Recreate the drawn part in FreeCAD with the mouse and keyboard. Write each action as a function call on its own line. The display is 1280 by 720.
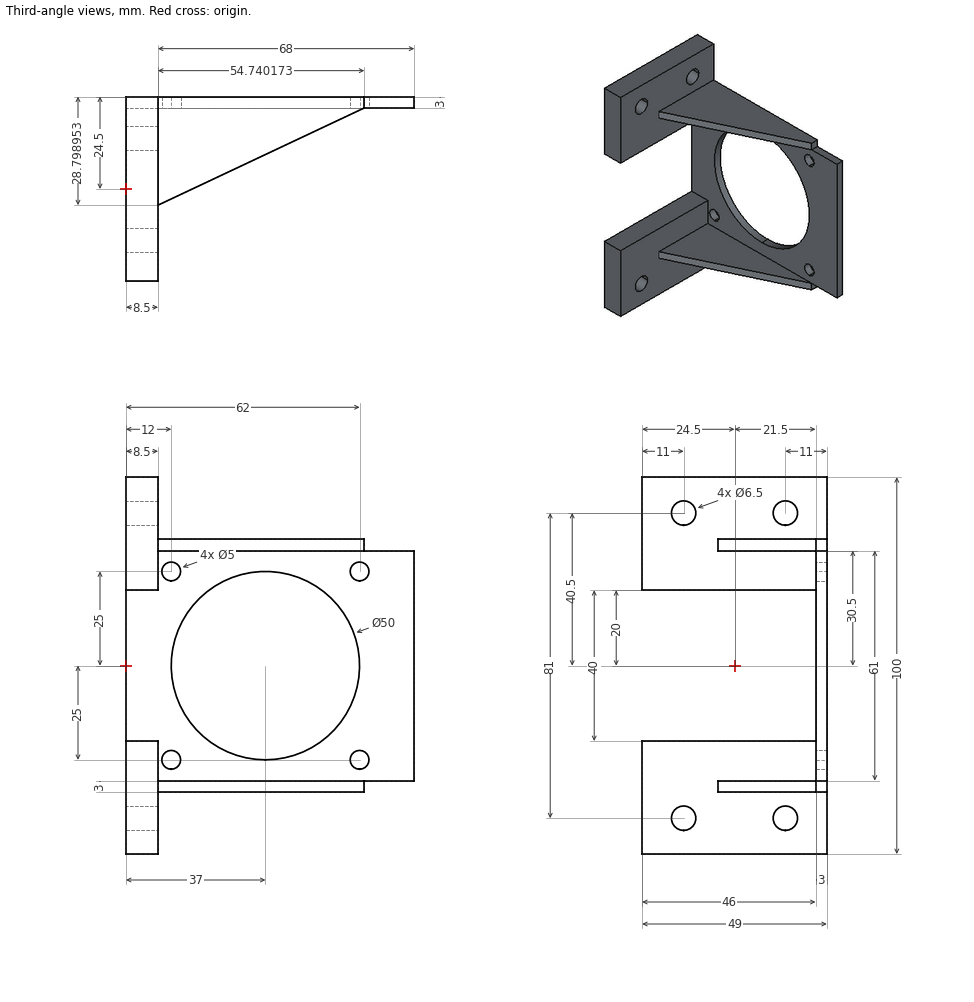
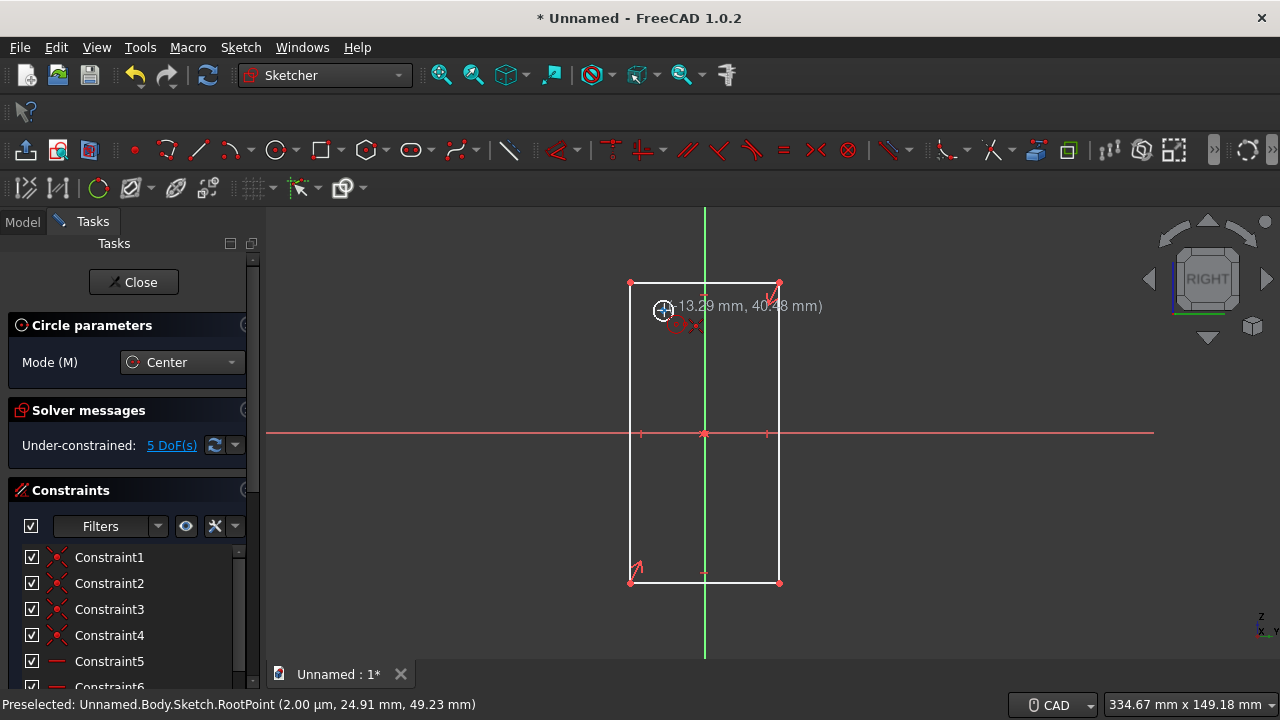
scroll(664, 556, up, 5)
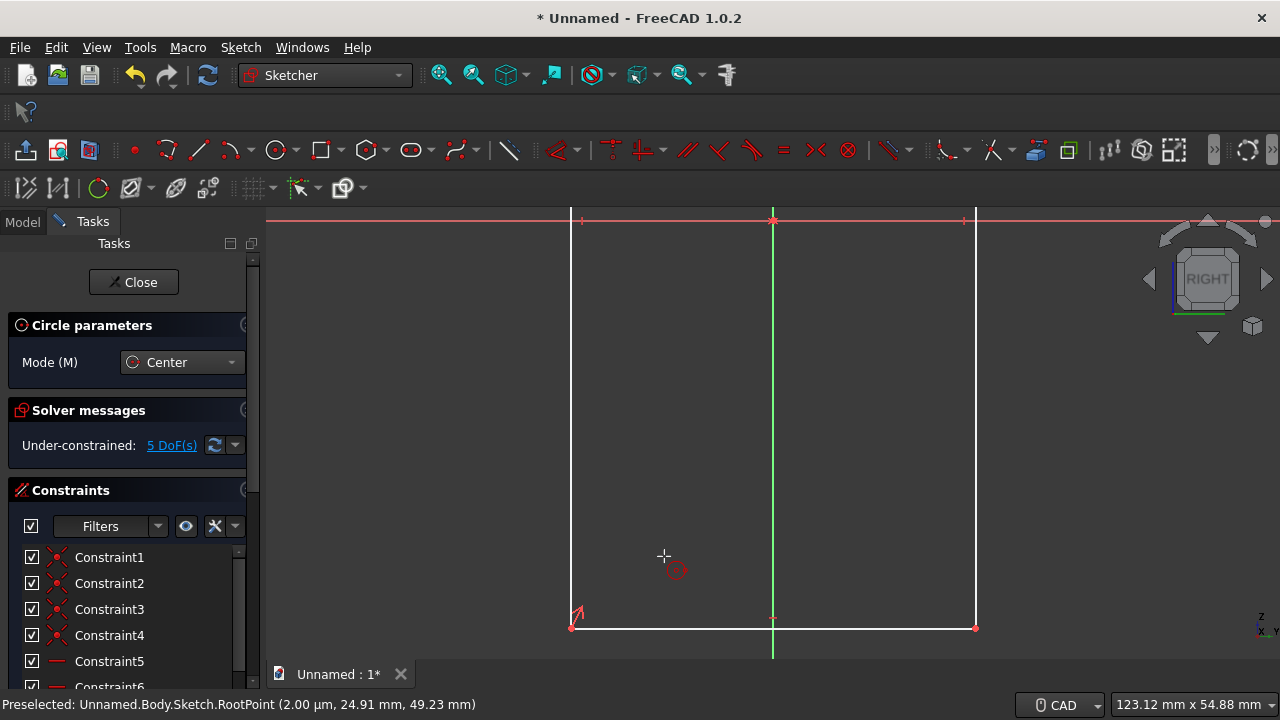
click(662, 554)
click(681, 535)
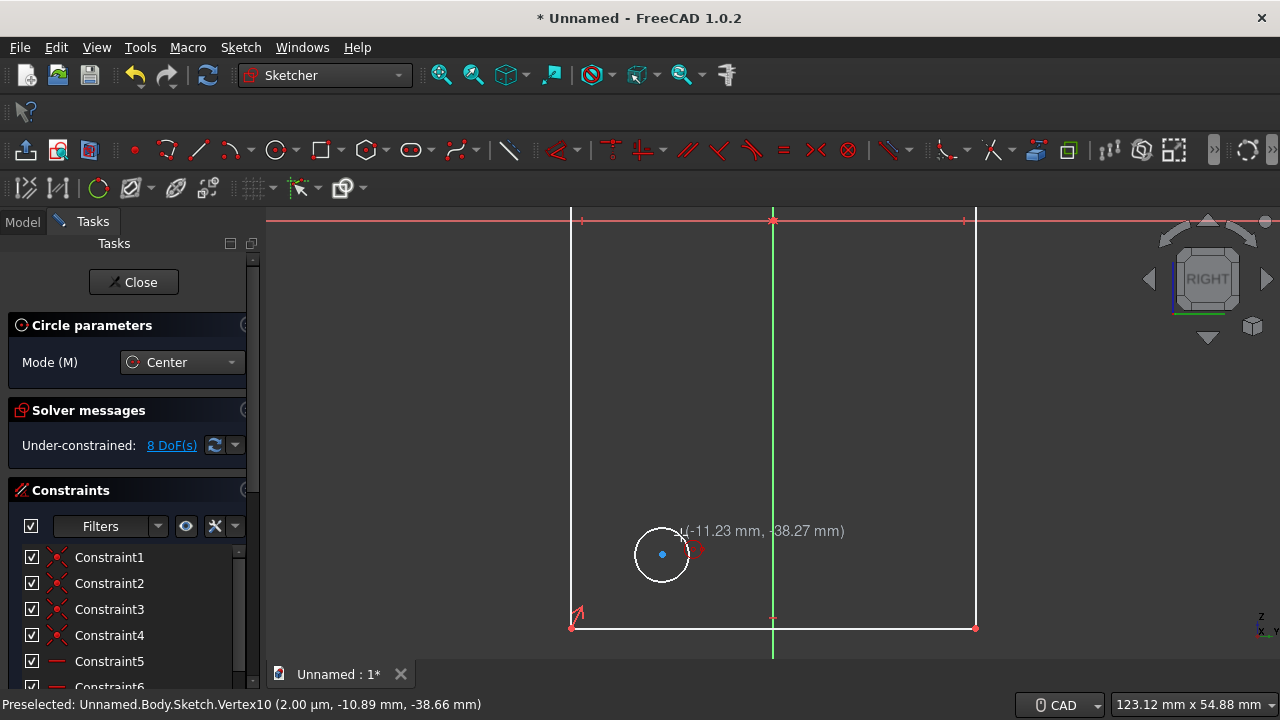
scroll(664, 557, down, 5)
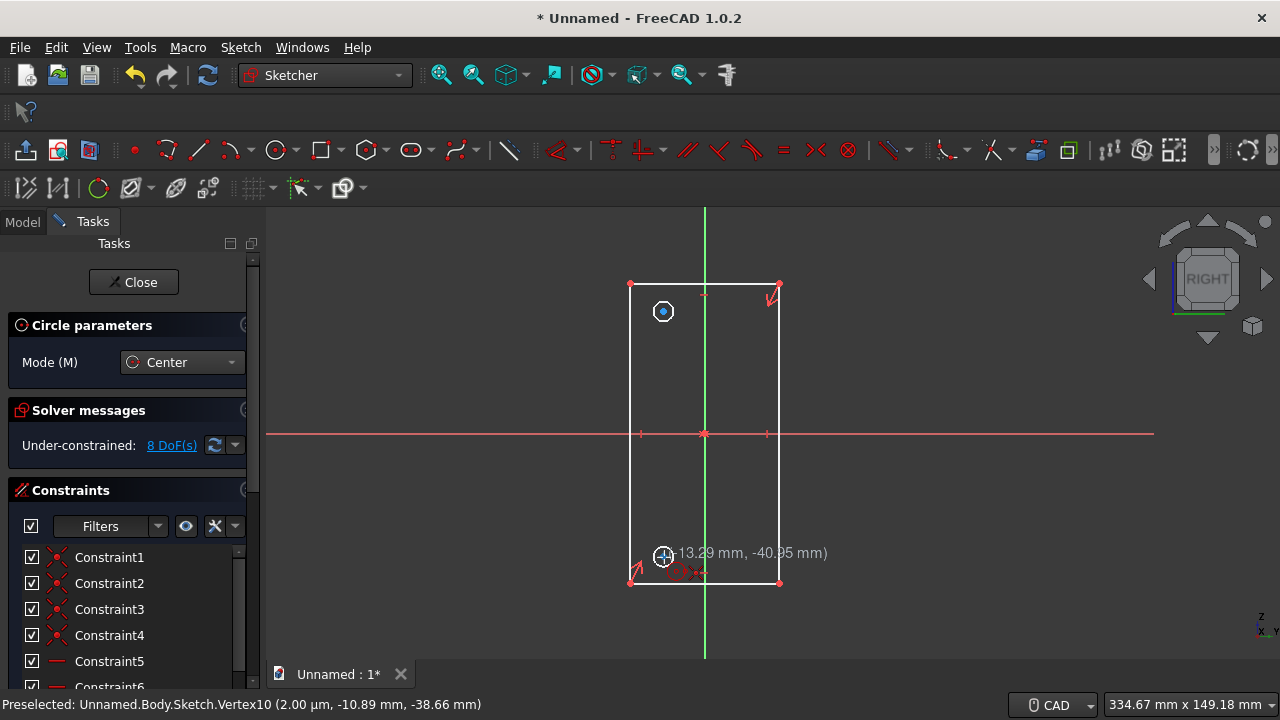
scroll(745, 311, up, 5)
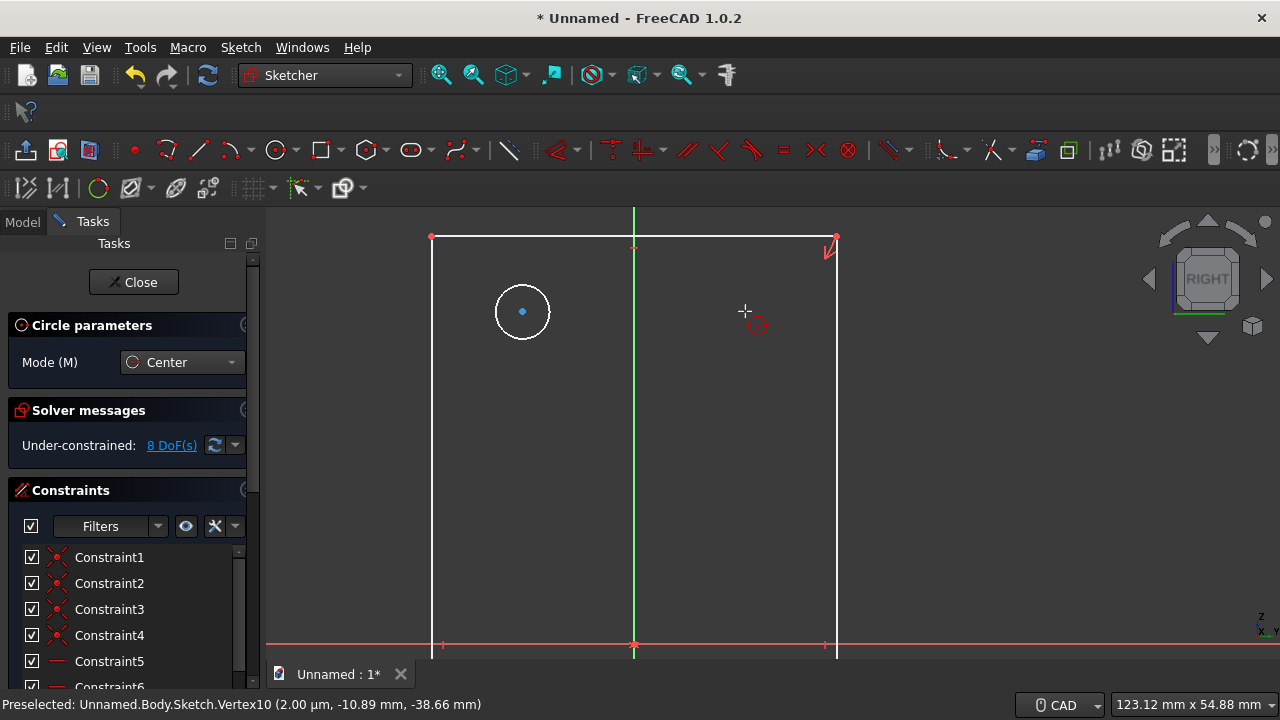
click(745, 311)
click(764, 292)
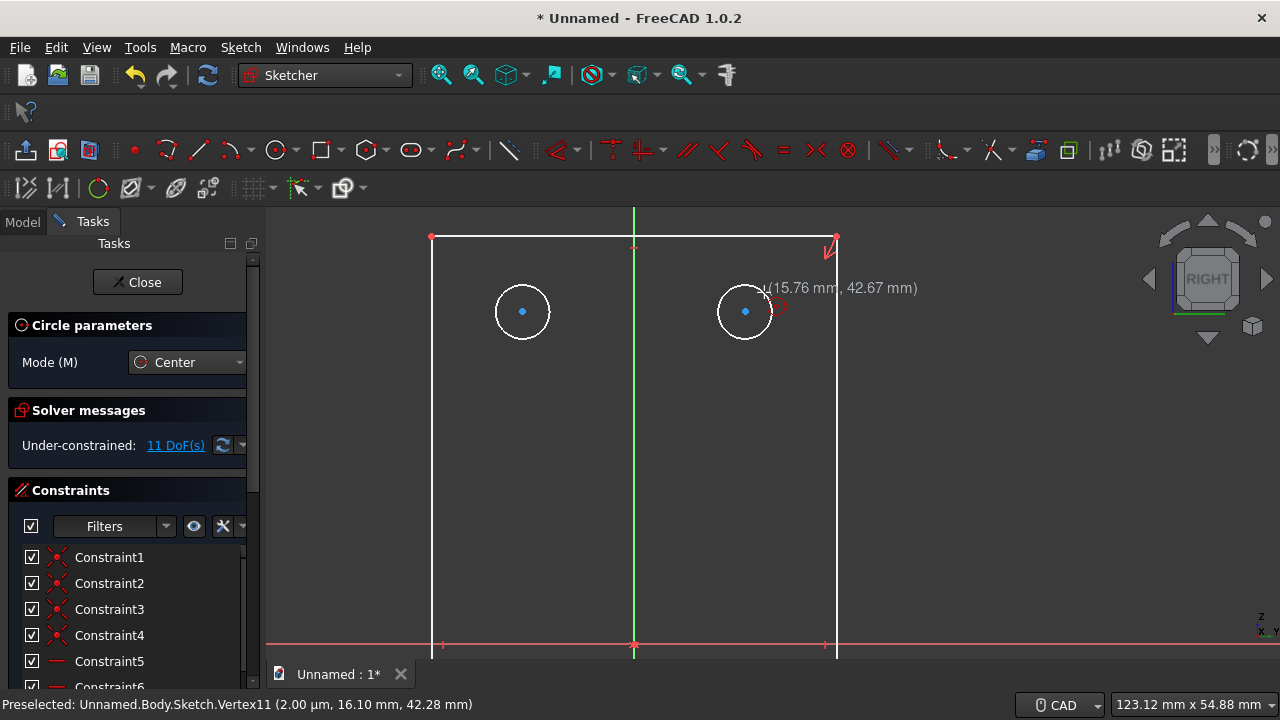
scroll(745, 310, down, 5)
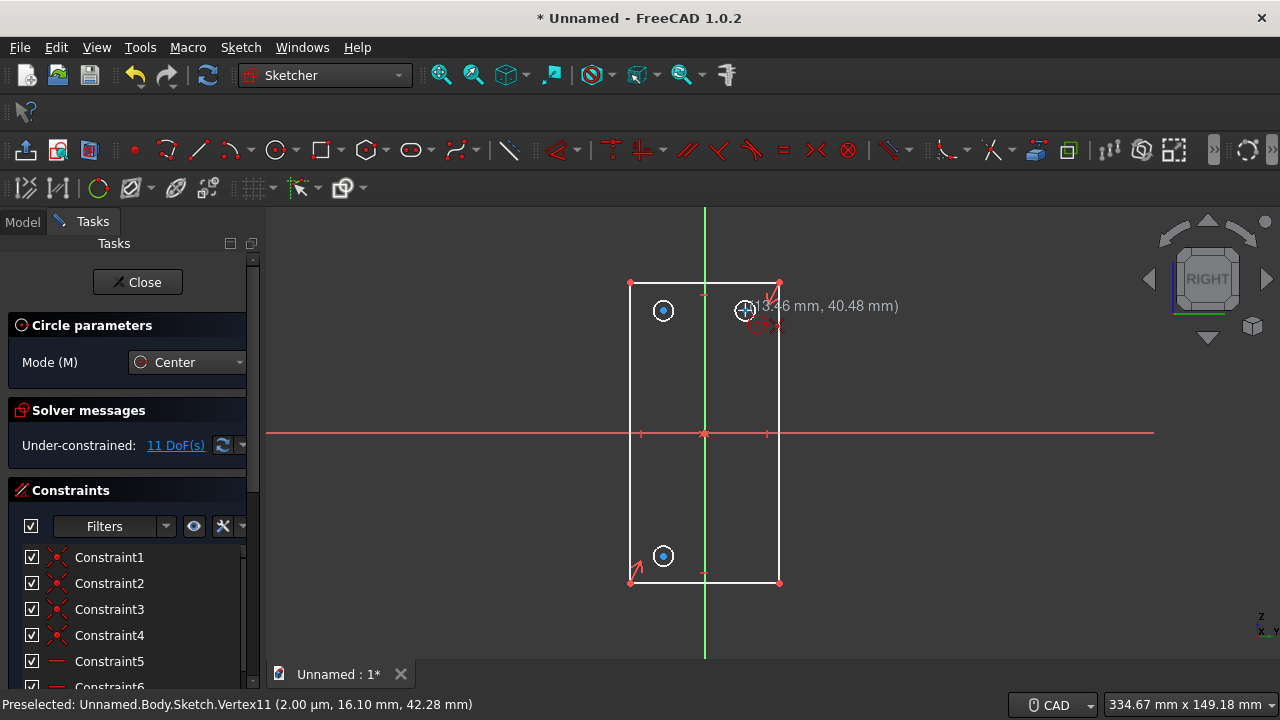
scroll(745, 556, up, 5)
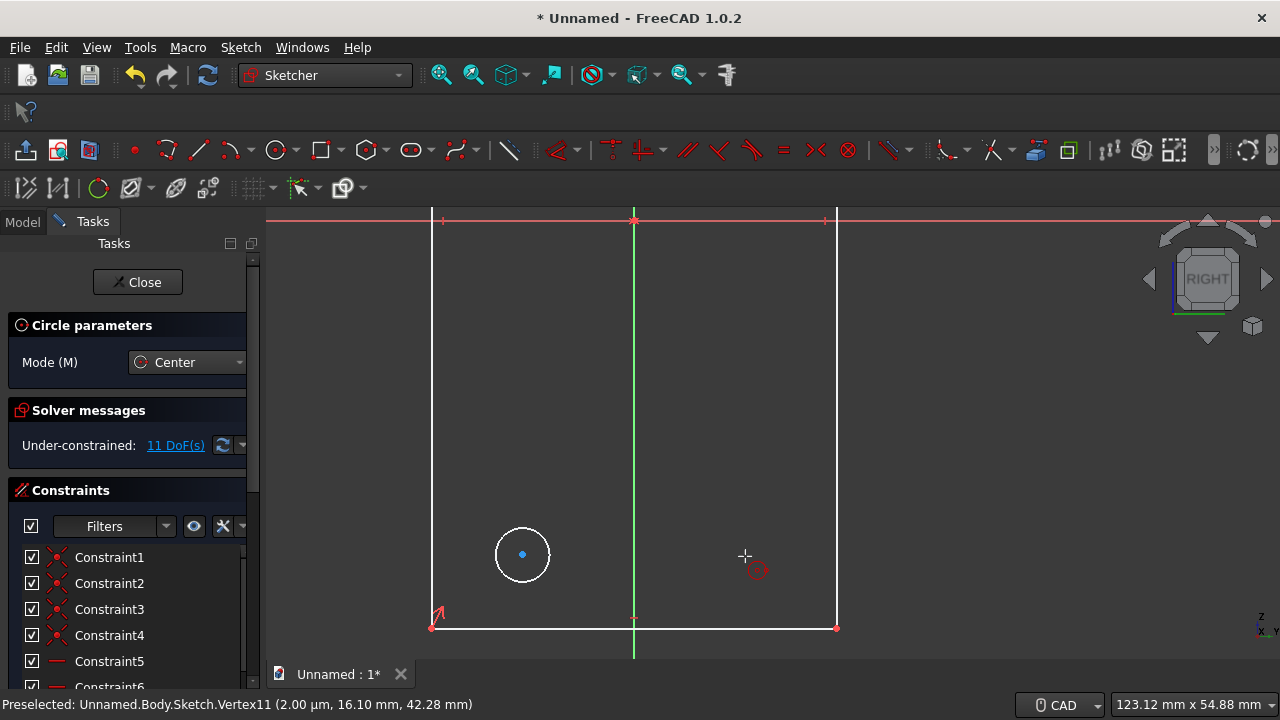
click(745, 554)
click(764, 535)
key(Escape)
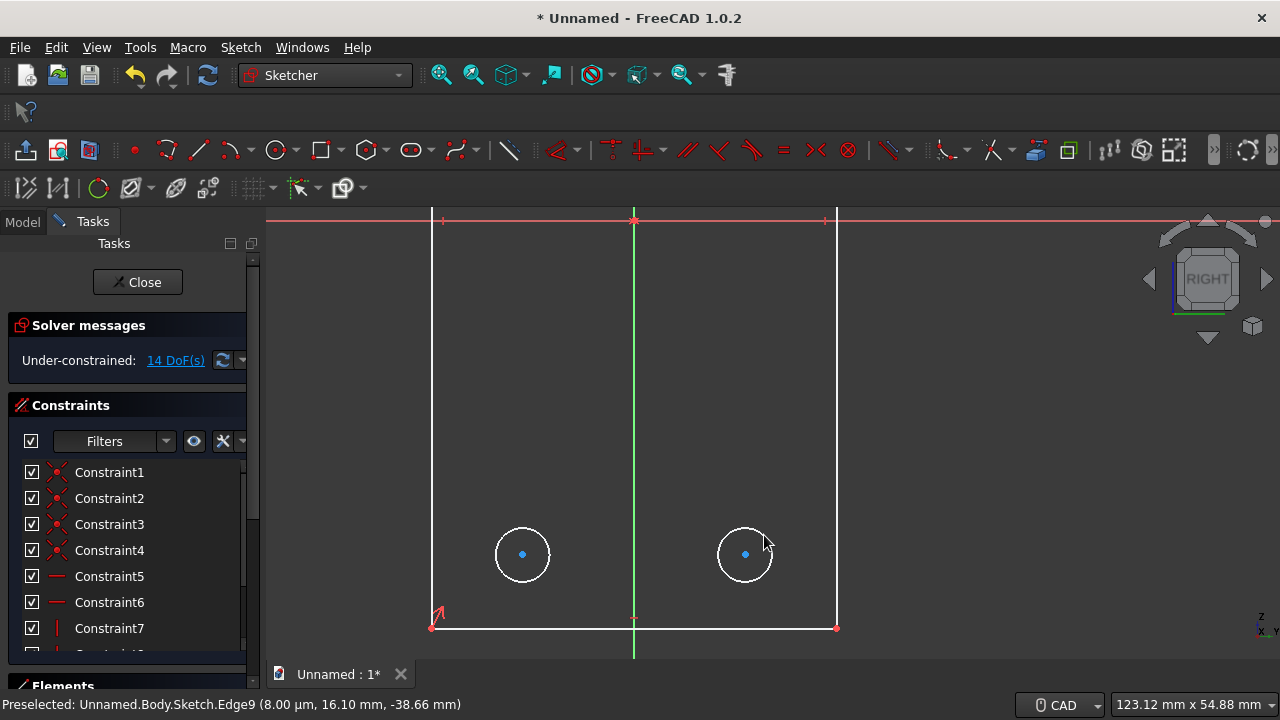
scroll(745, 557, down, 5)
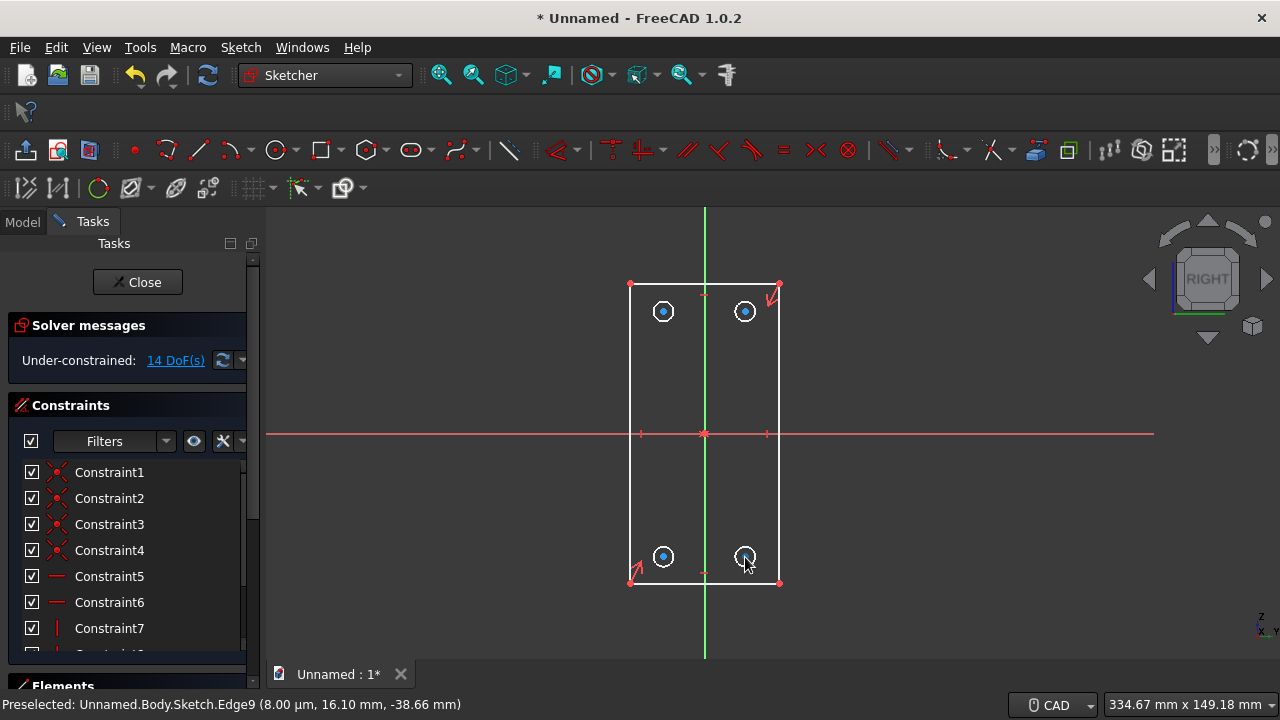
scroll(670, 305, up, 2)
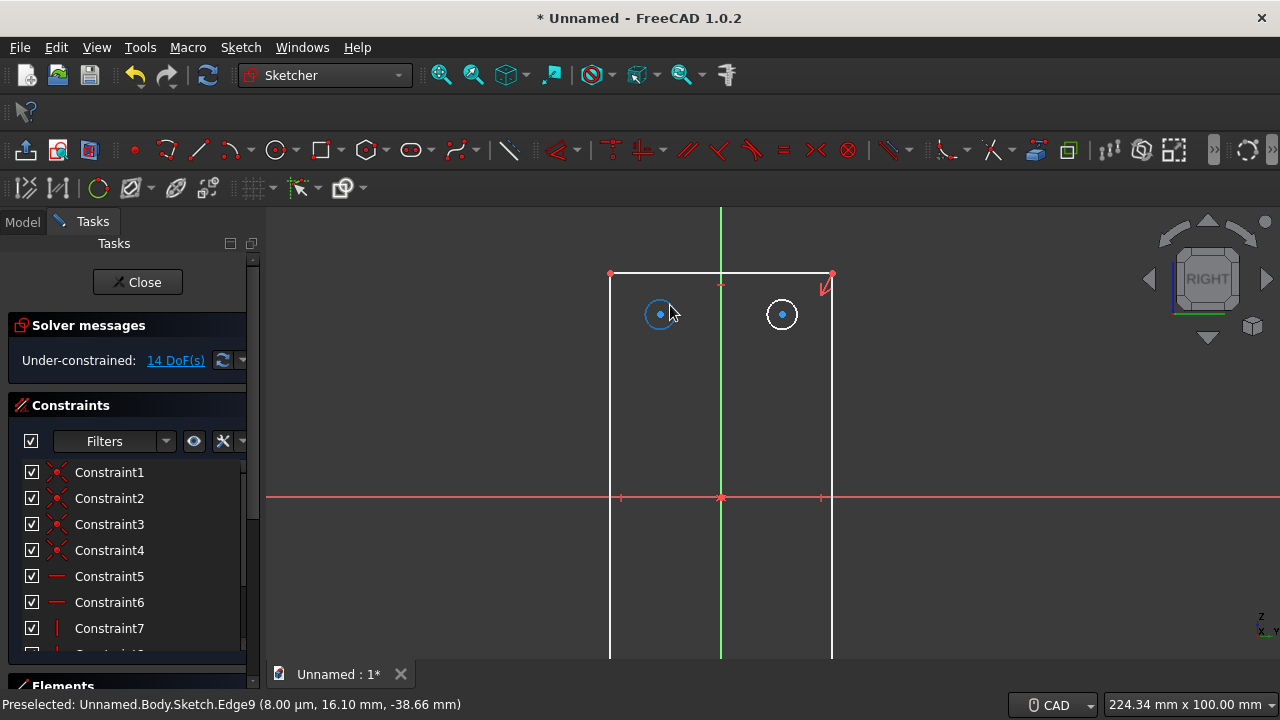
click(671, 304)